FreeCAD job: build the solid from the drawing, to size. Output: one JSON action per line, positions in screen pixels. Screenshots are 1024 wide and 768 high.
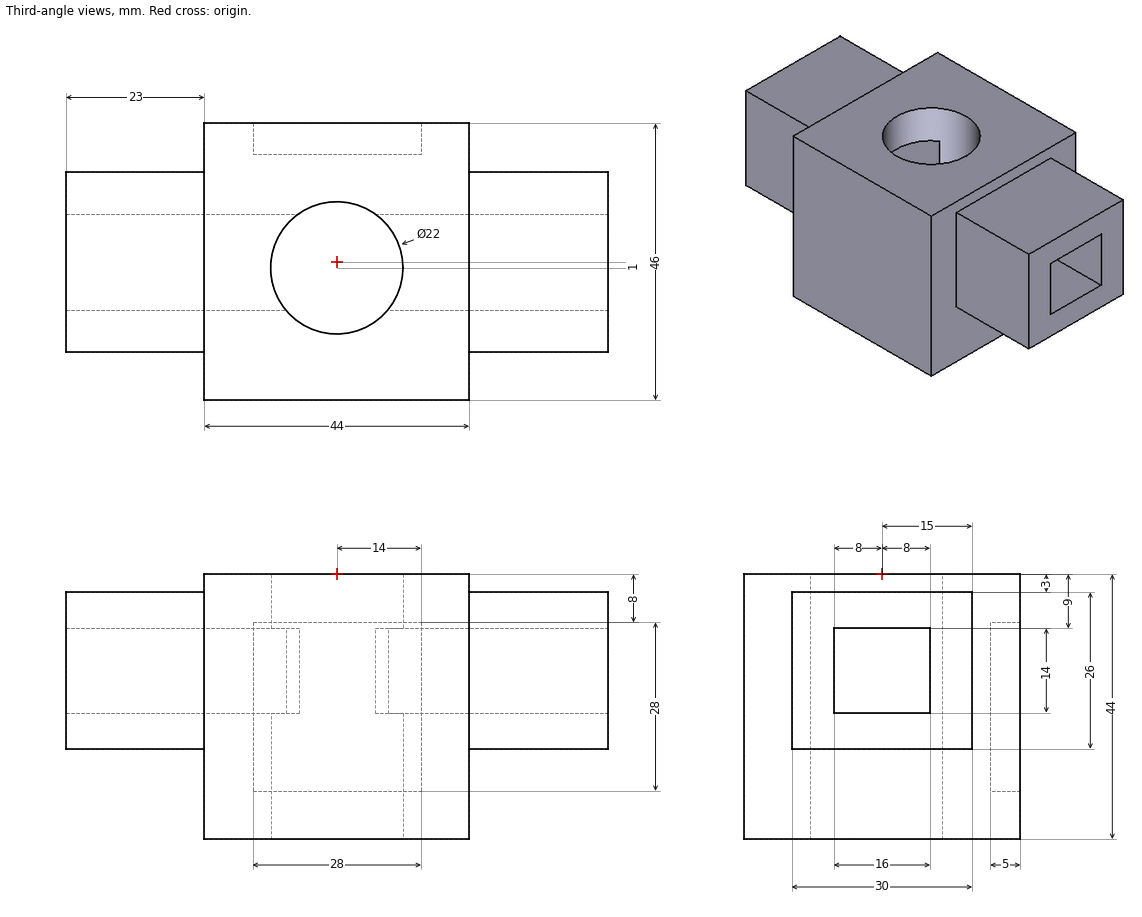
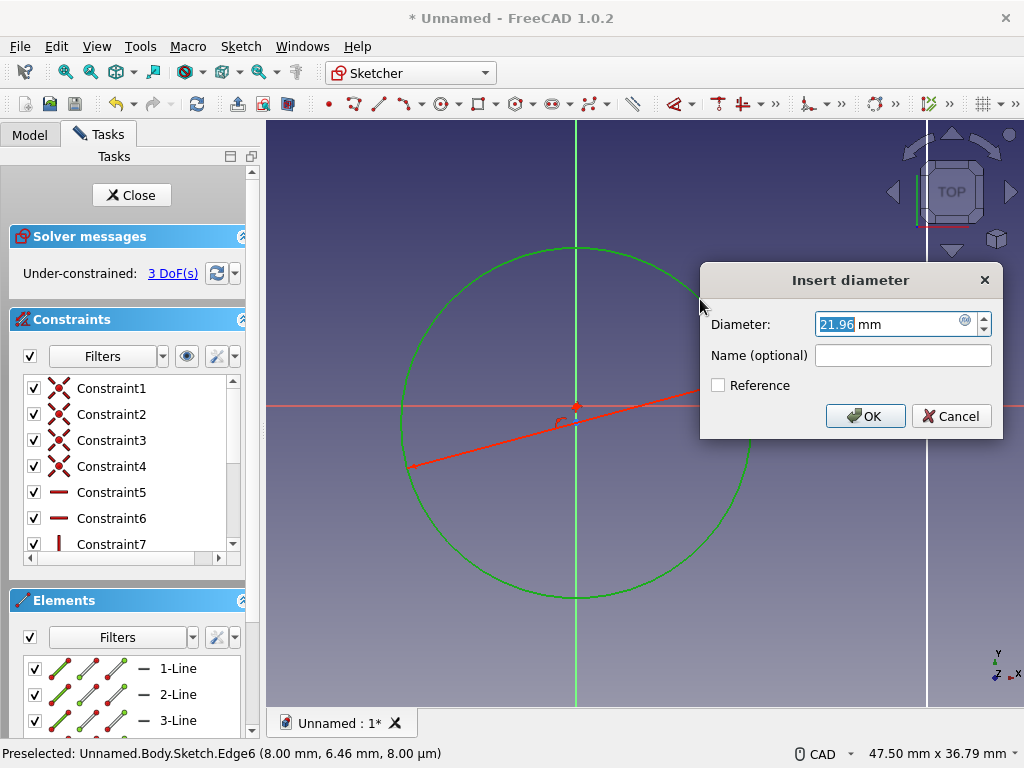
{"action": "type", "text": "22"}
{"action": "key", "text": "Return"}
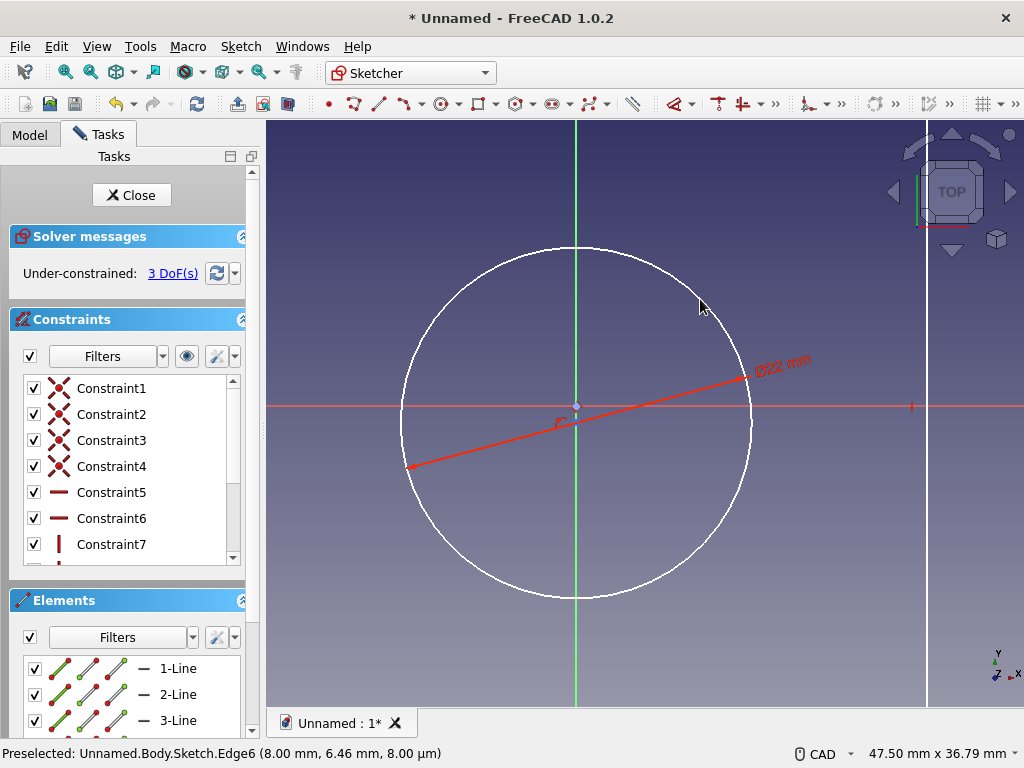
{"action": "scroll", "coordinate": [576, 423], "scroll_direction": "up", "scroll_amount": 5}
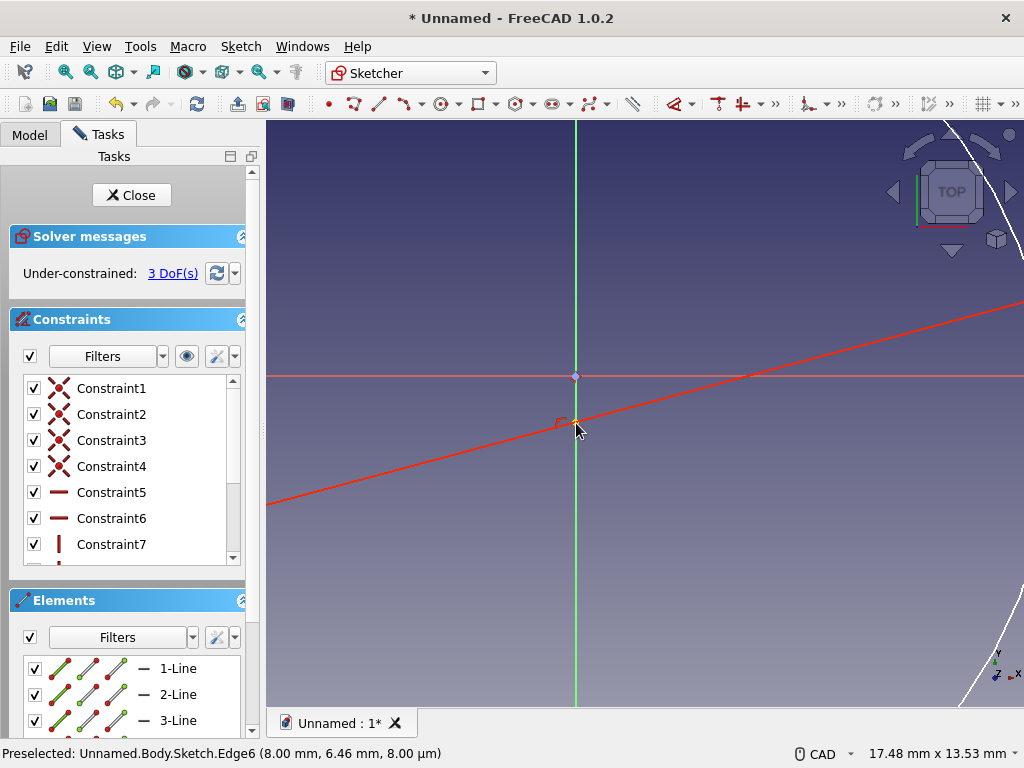
{"action": "left_click", "coordinate": [576, 422]}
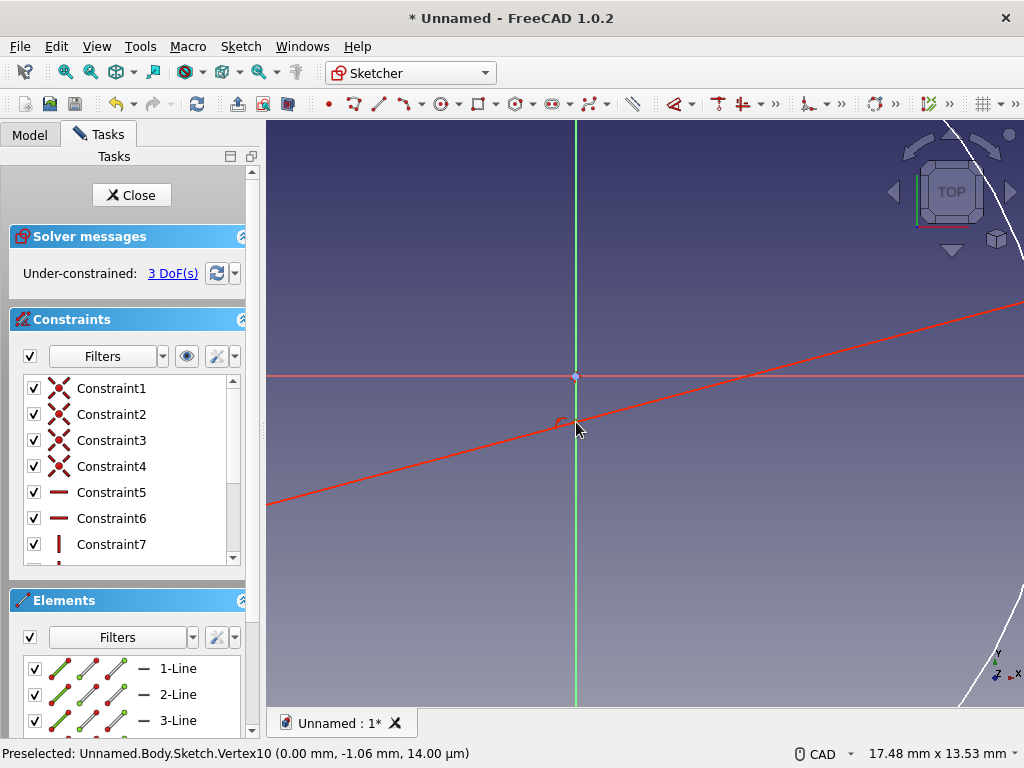
{"action": "key", "text": "i"}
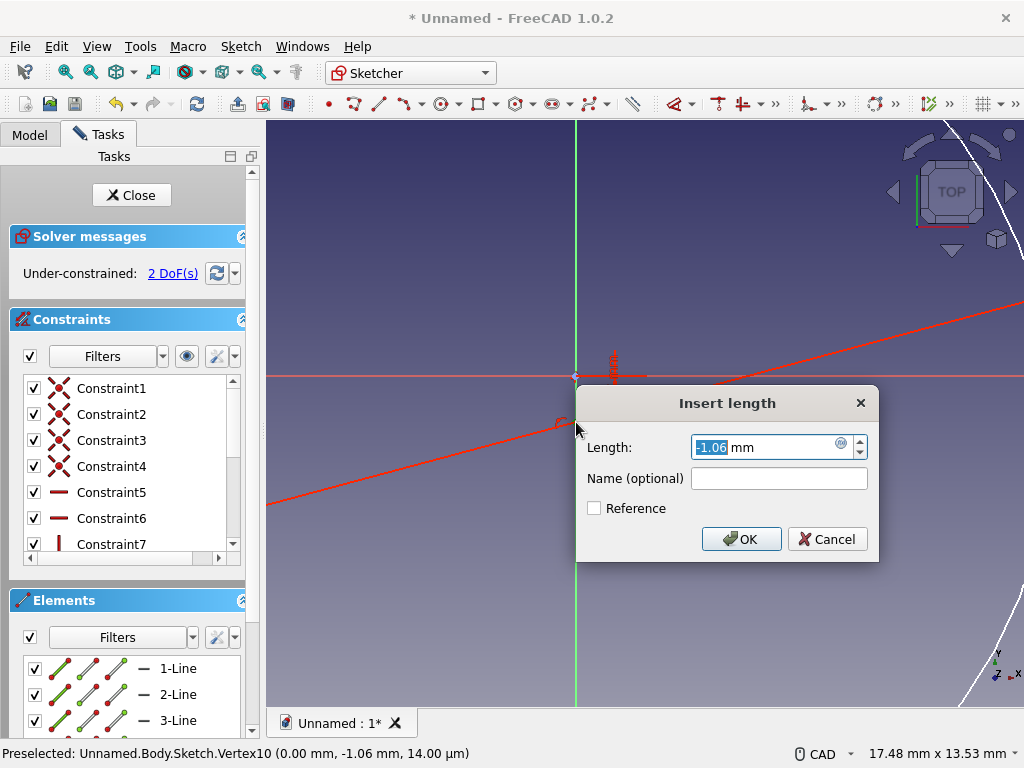
{"action": "type", "text": "-1"}
{"action": "key", "text": "Return"}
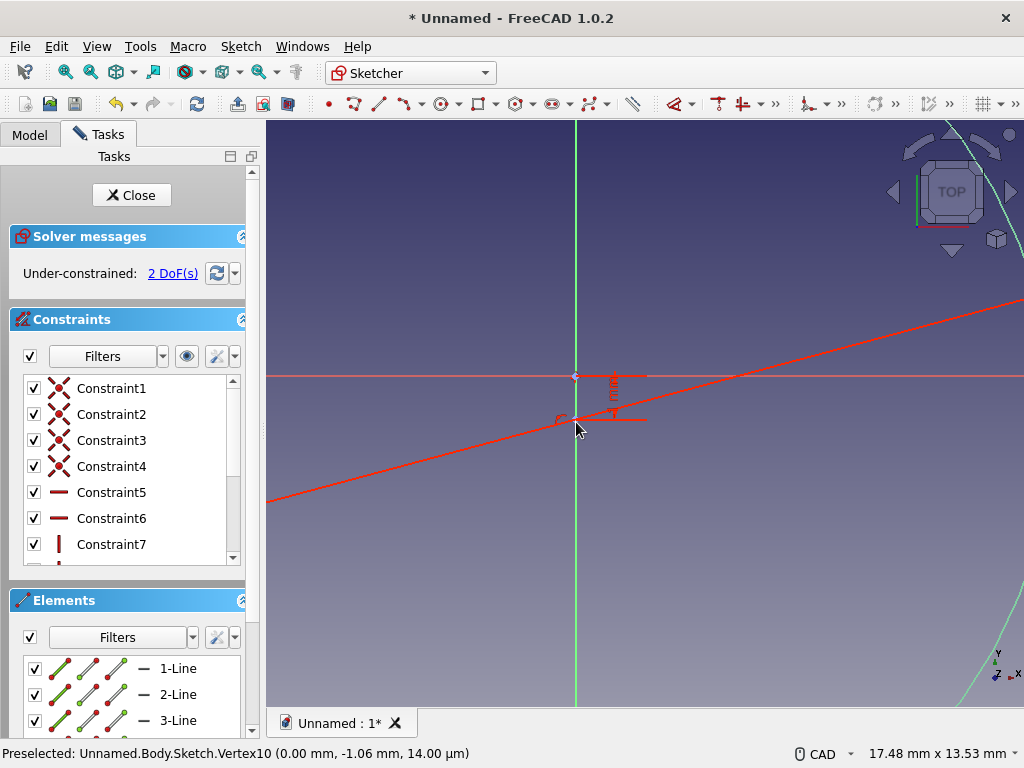
{"action": "scroll", "coordinate": [577, 423], "scroll_direction": "down", "scroll_amount": 8}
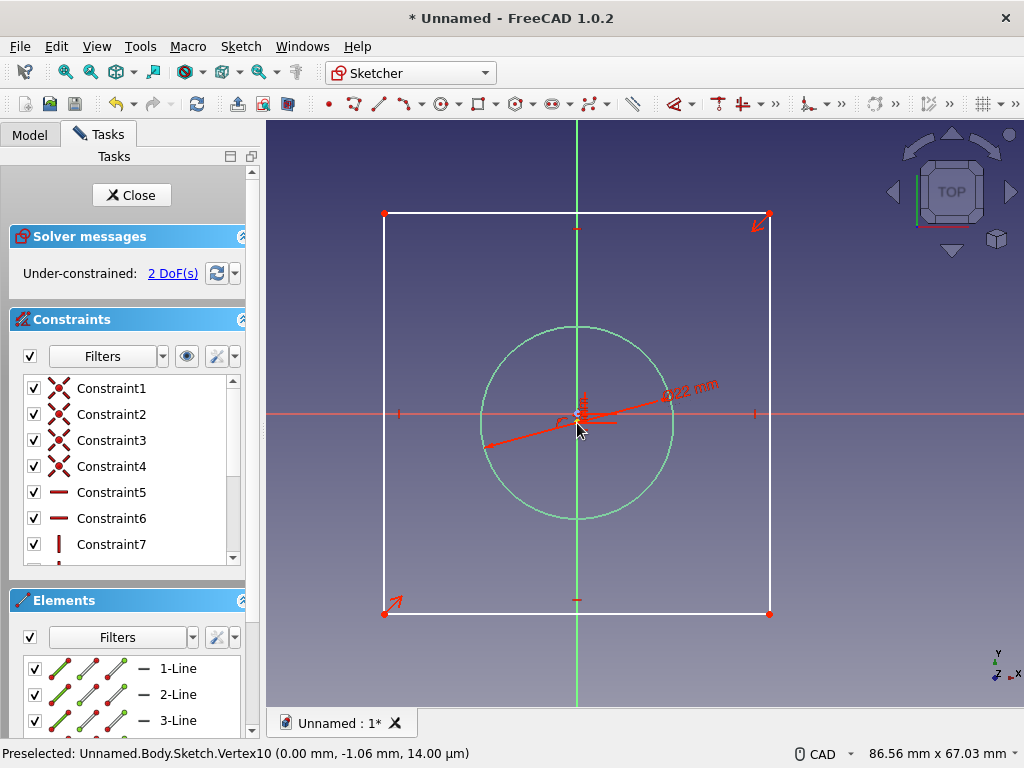
{"action": "left_click", "coordinate": [500, 614]}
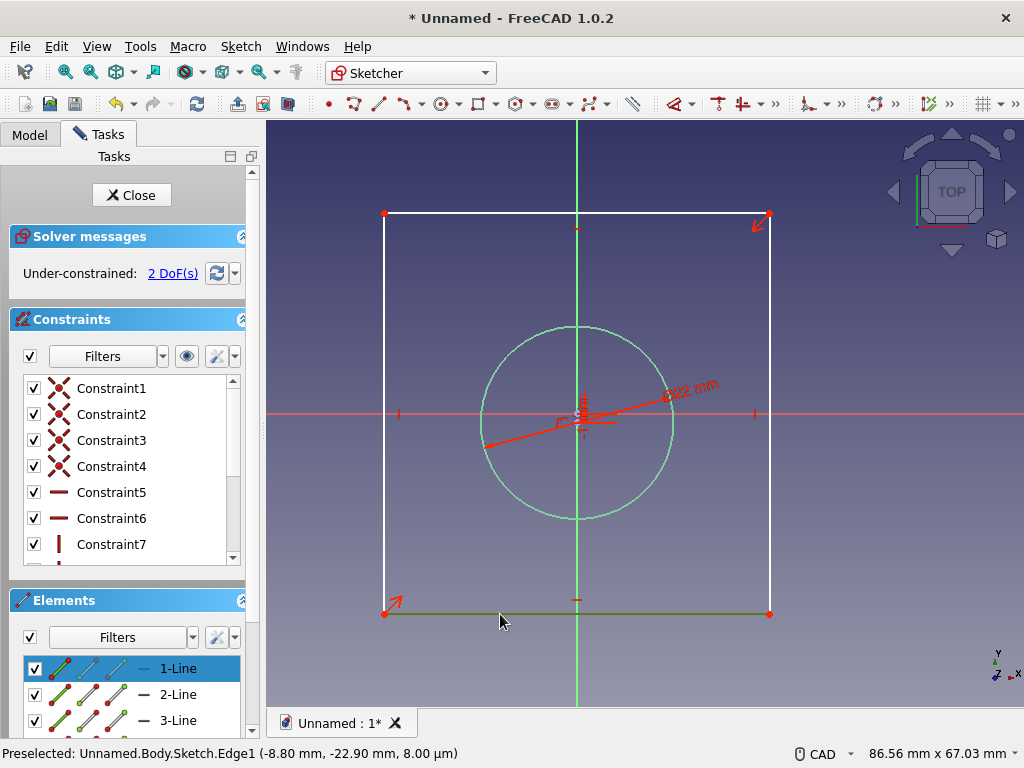
{"action": "key", "text": "l"}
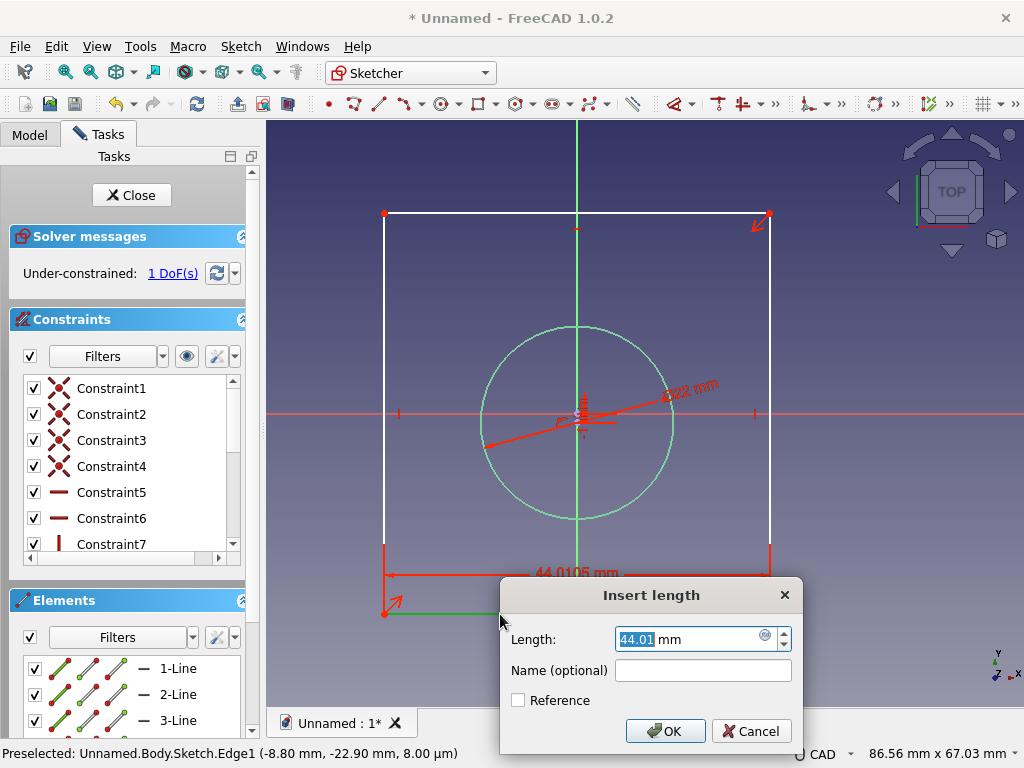
{"action": "type", "text": "44"}
{"action": "key", "text": "Return"}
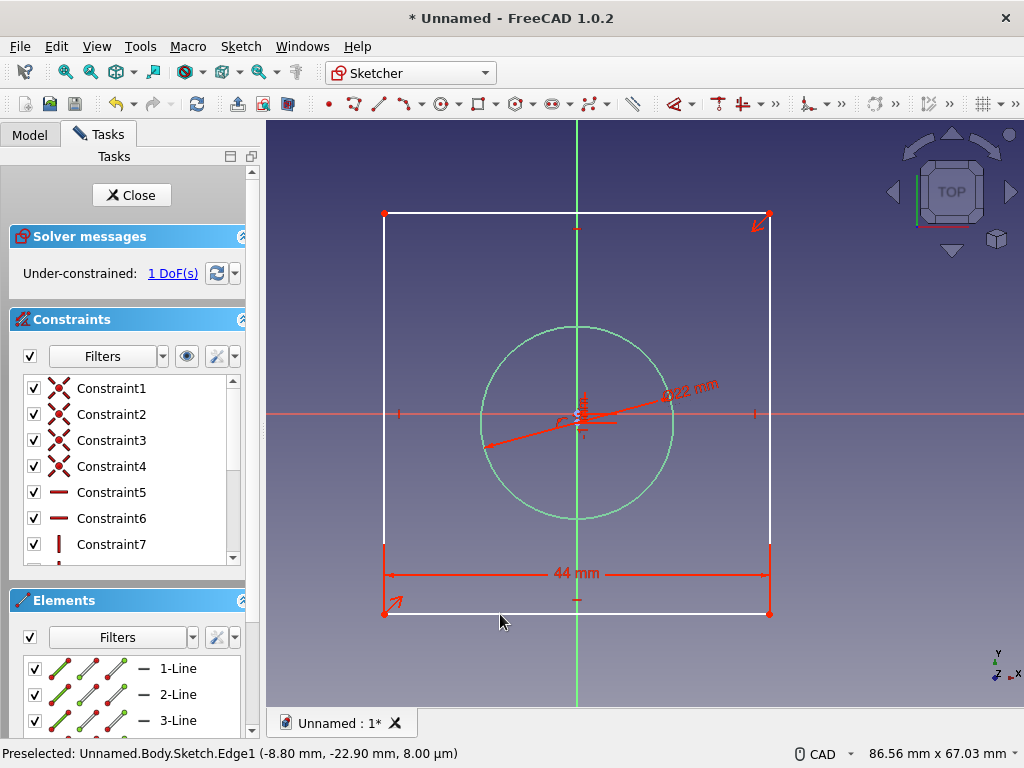
{"action": "left_click", "coordinate": [770, 494]}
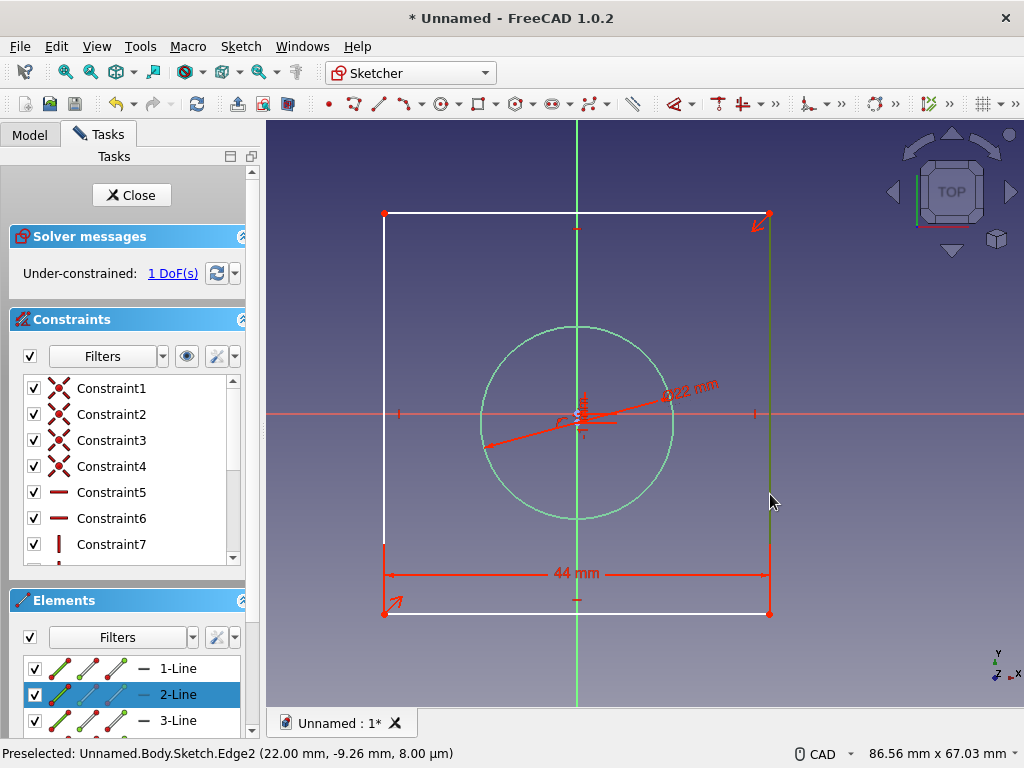
{"action": "key", "text": "i"}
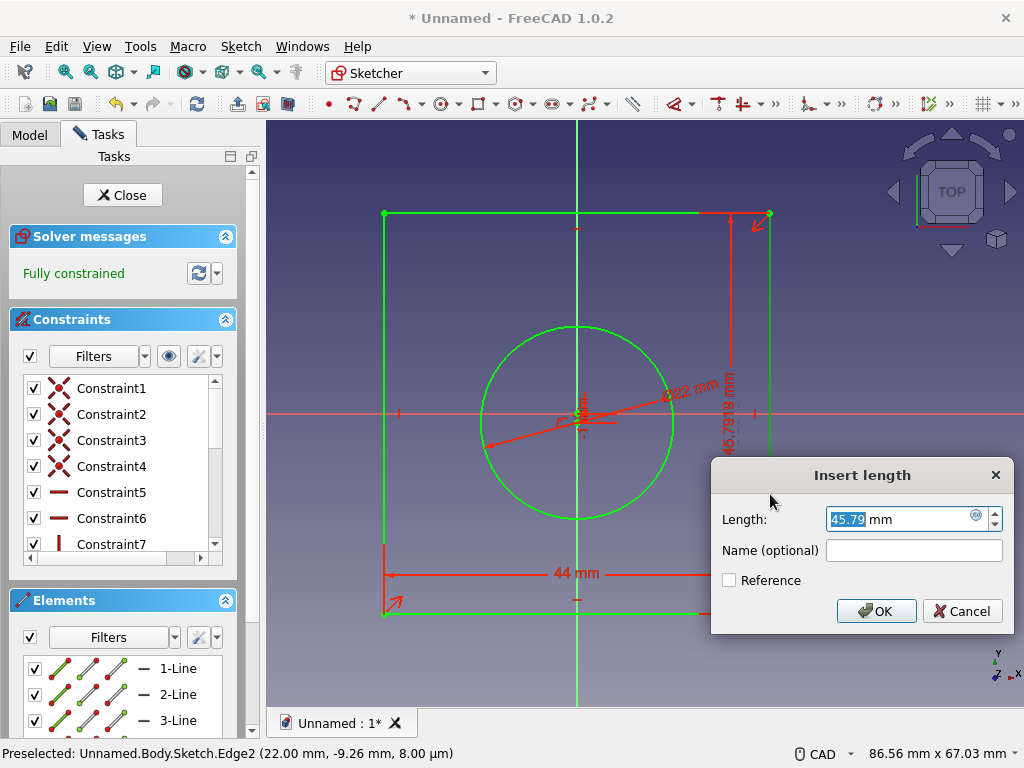
{"action": "type", "text": "46"}
{"action": "key", "text": "Return"}